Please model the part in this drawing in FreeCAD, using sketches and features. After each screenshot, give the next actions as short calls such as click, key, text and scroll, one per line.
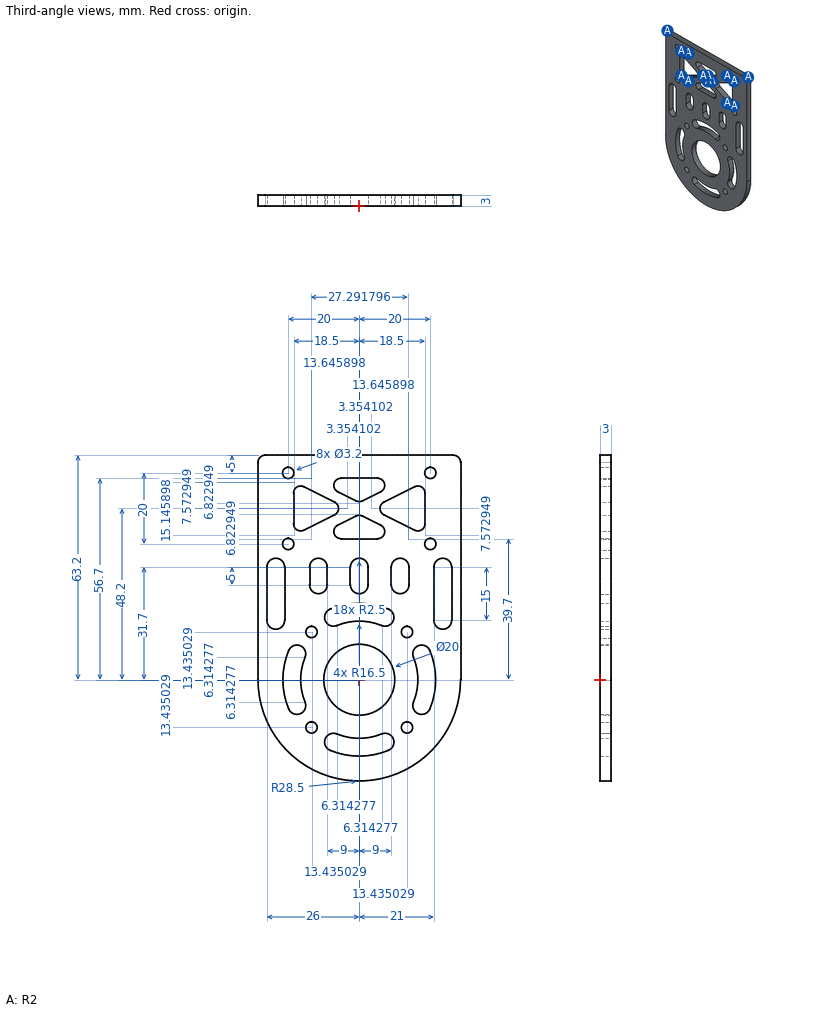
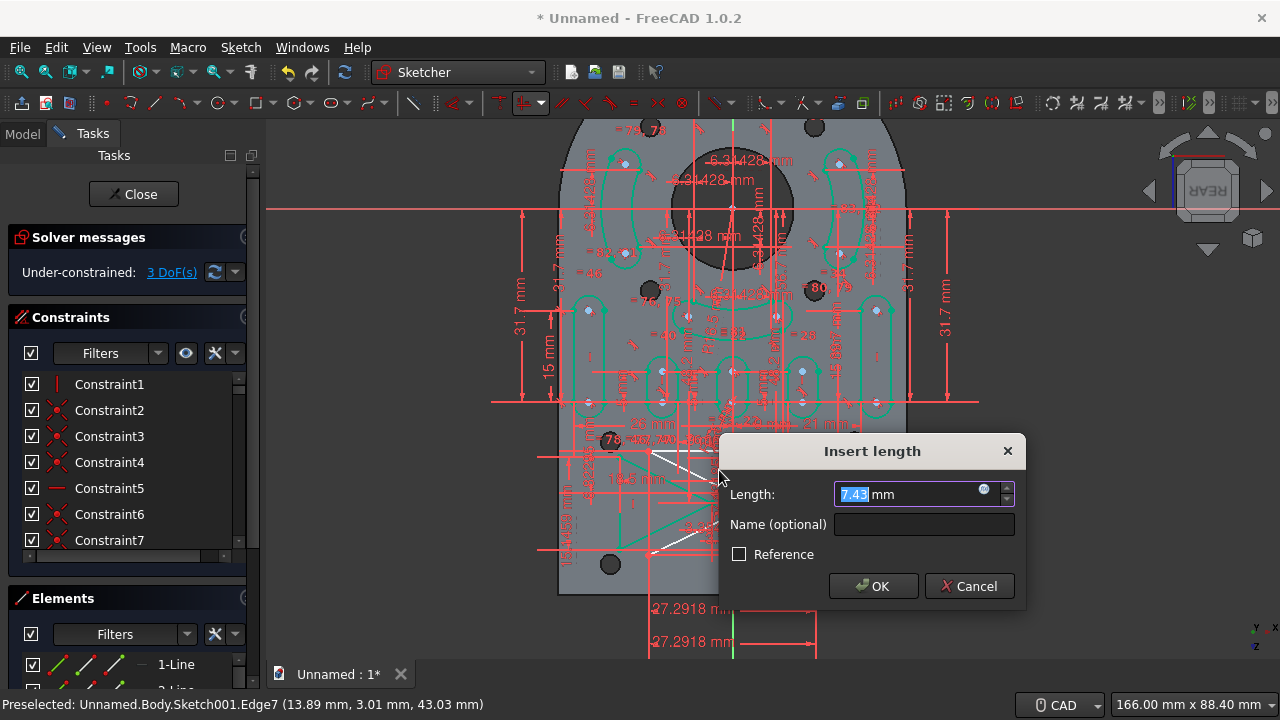
text(7.572949)
key(Return)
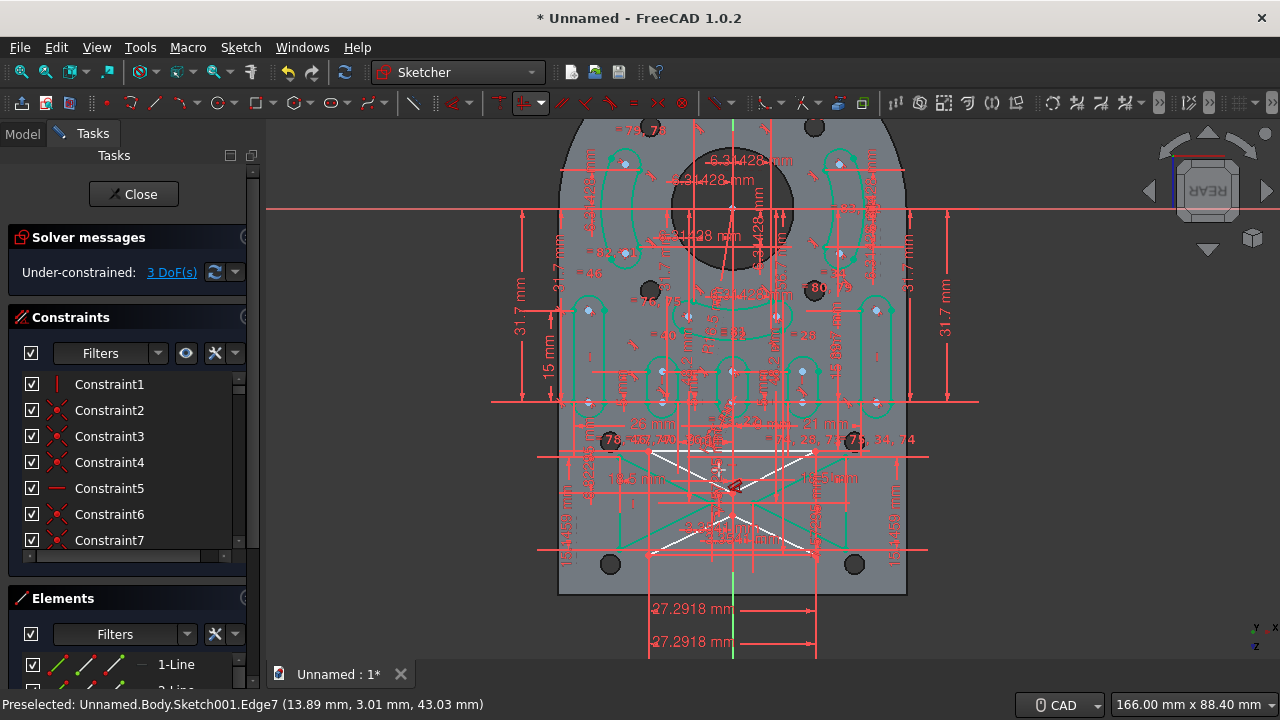
click(707, 527)
click(591, 549)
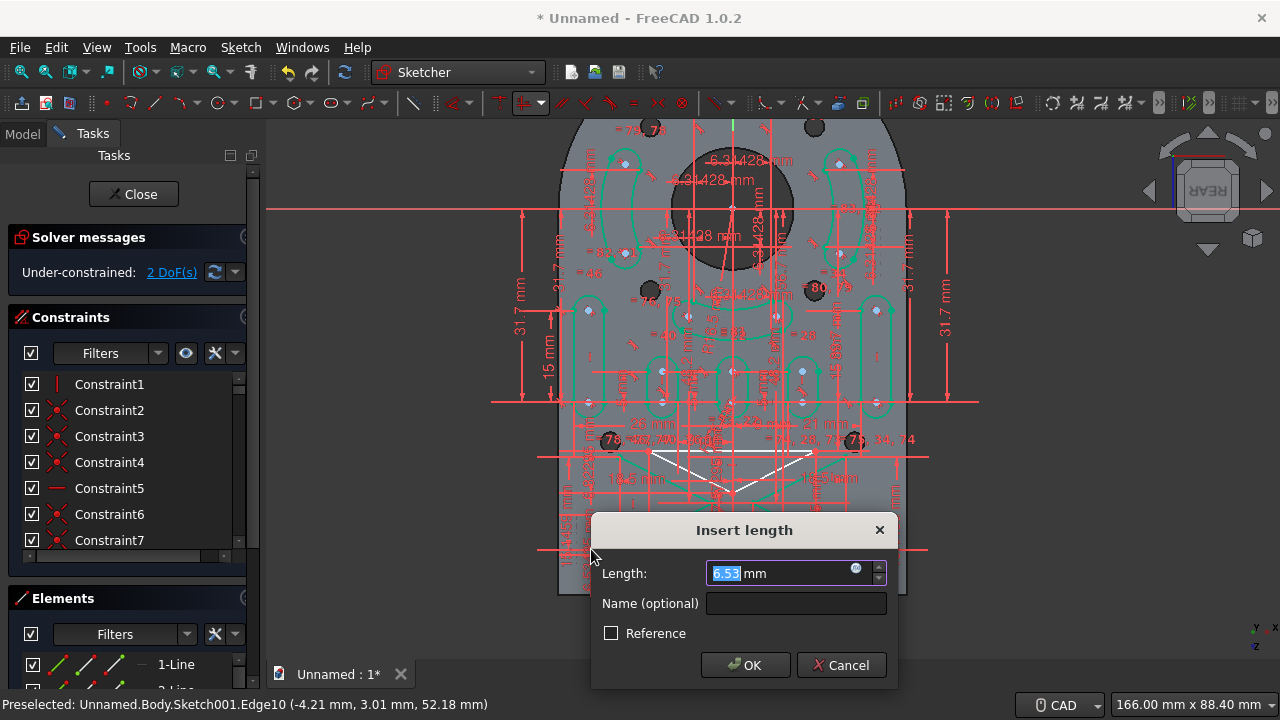
text(6.822949)
key(Return)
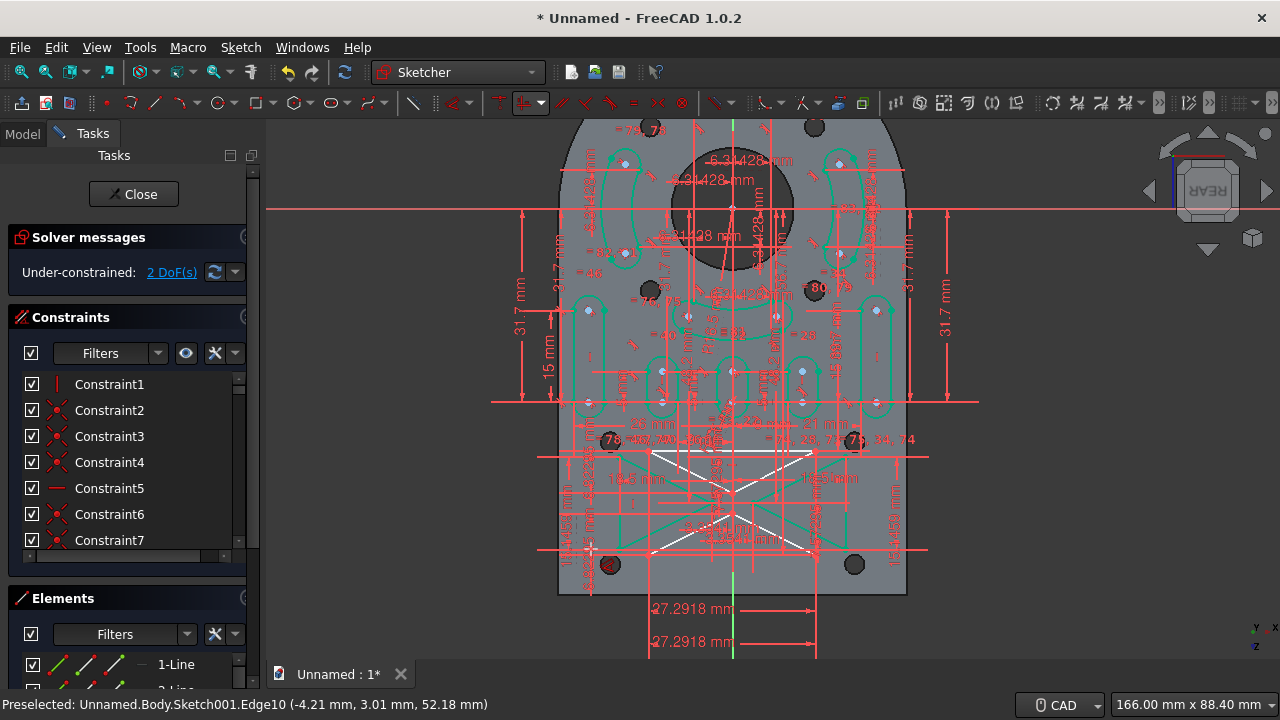
click(816, 451)
click(774, 581)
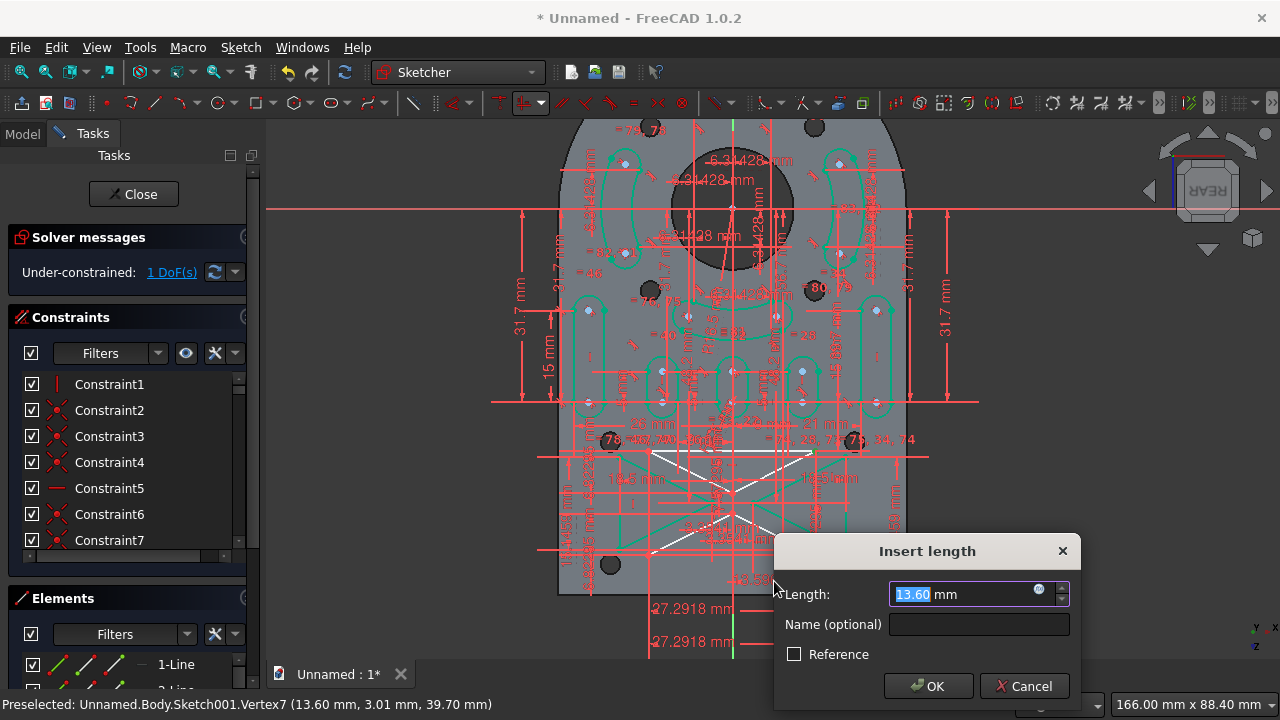
text(13.645898)
key(Return)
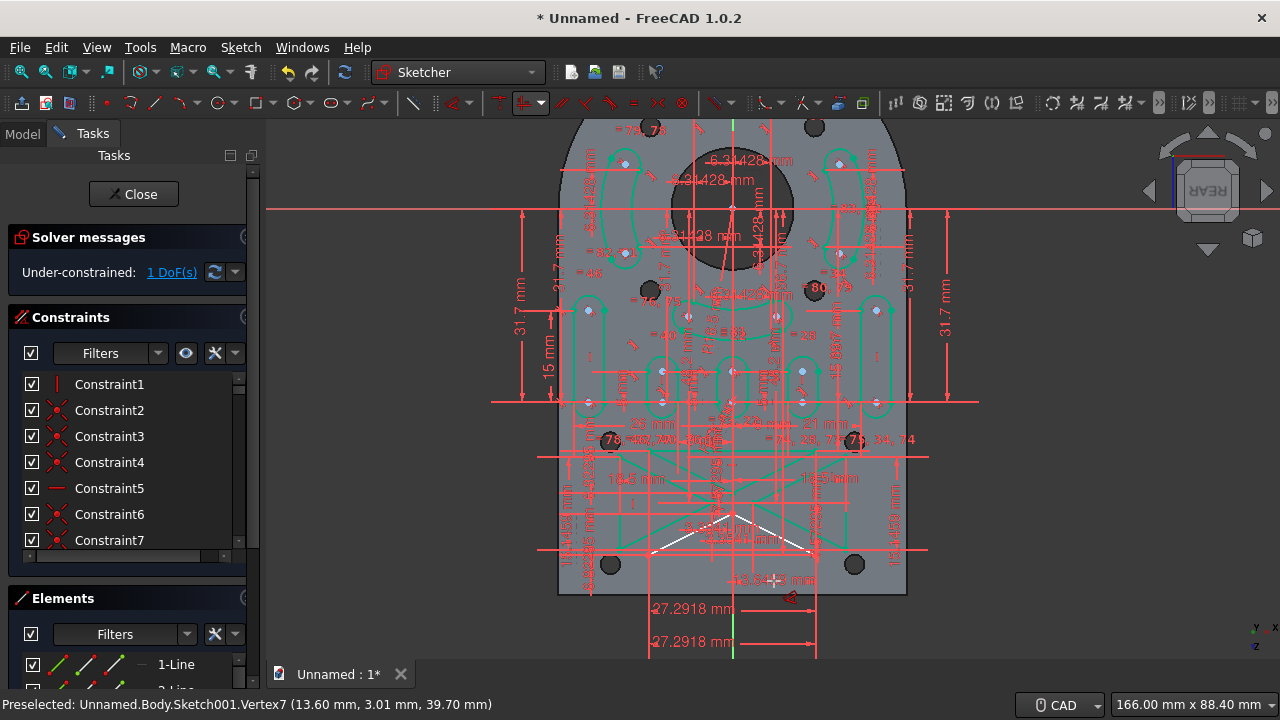
click(649, 555)
click(691, 589)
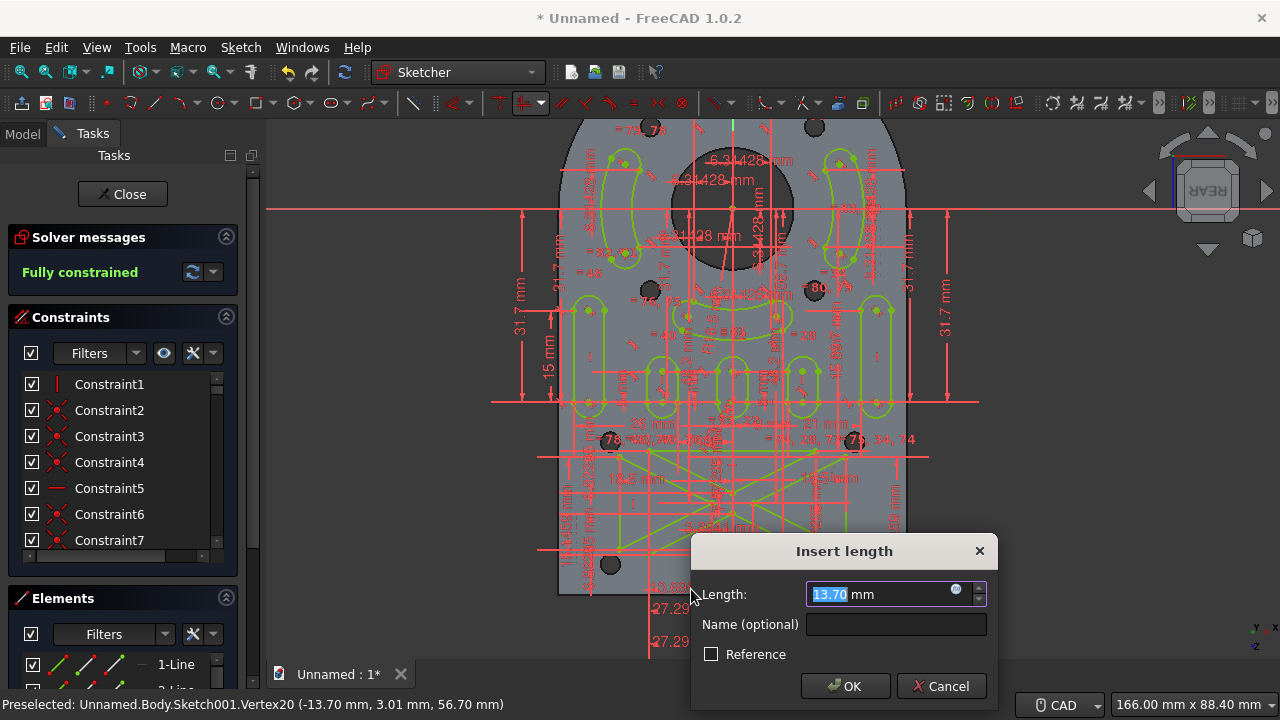
text(13.645898)
key(Return)
key(Escape)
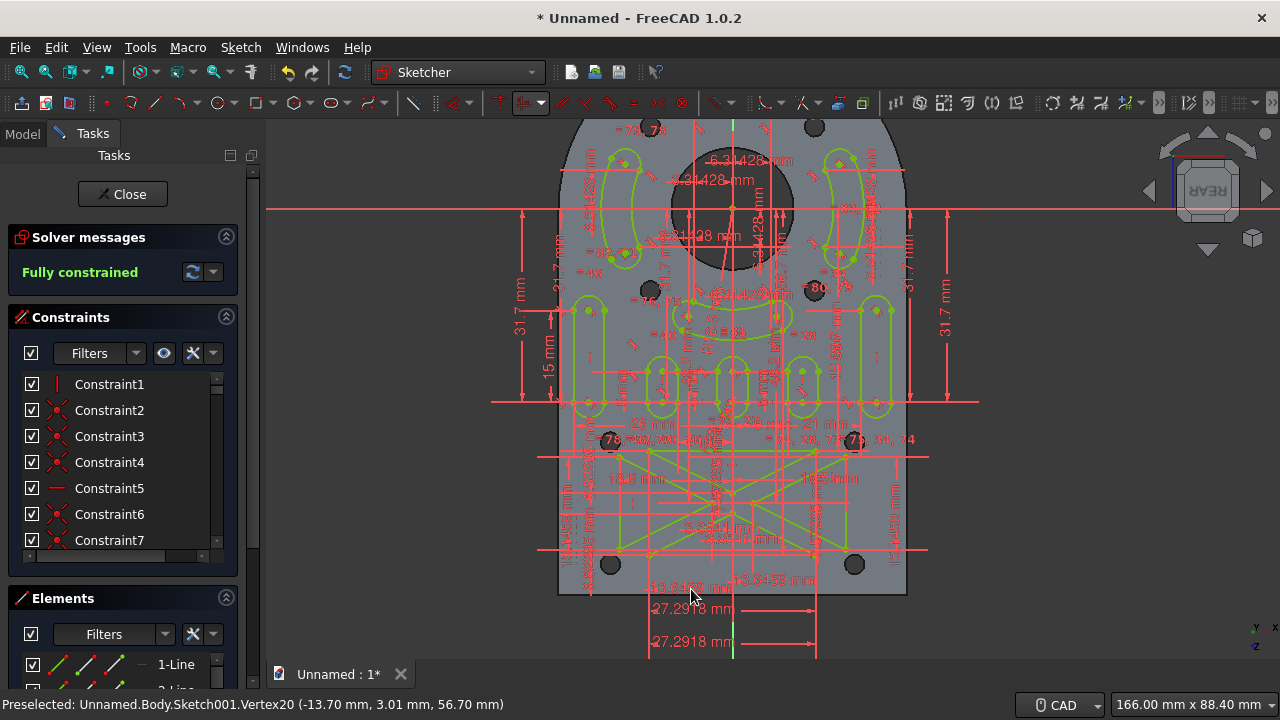
click(123, 194)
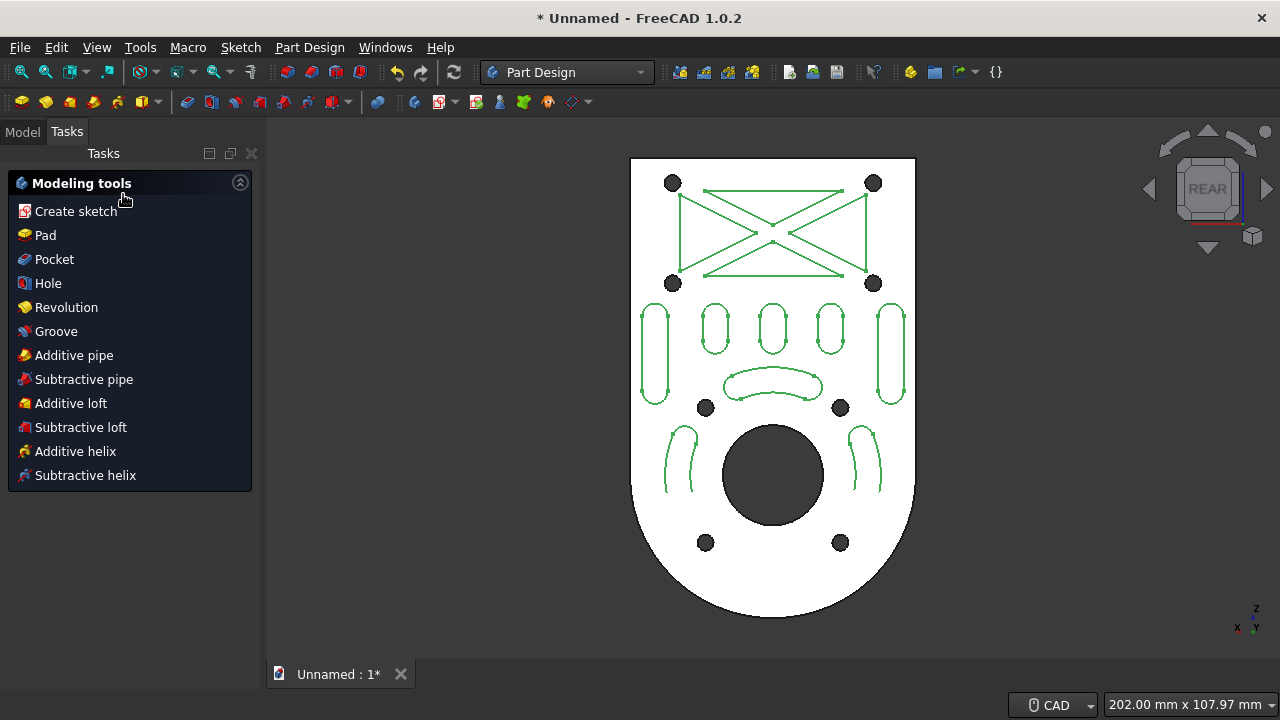
click(188, 102)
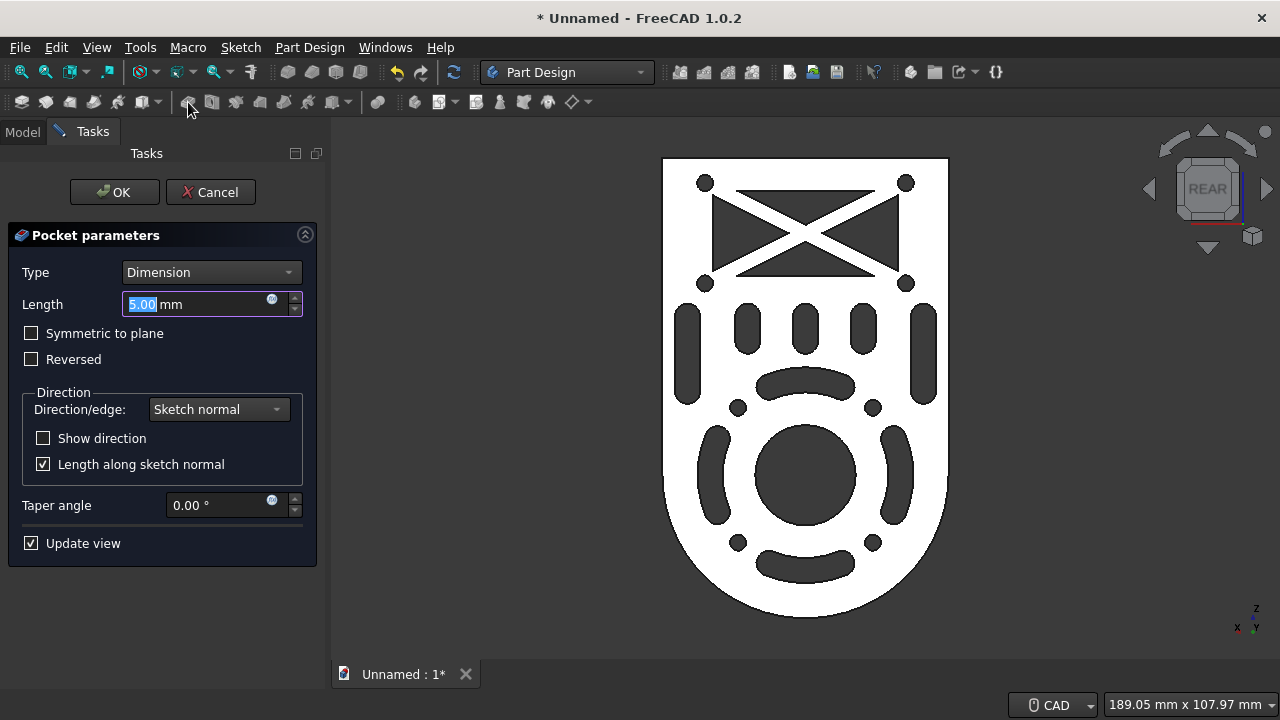
text(3)
key(Tab)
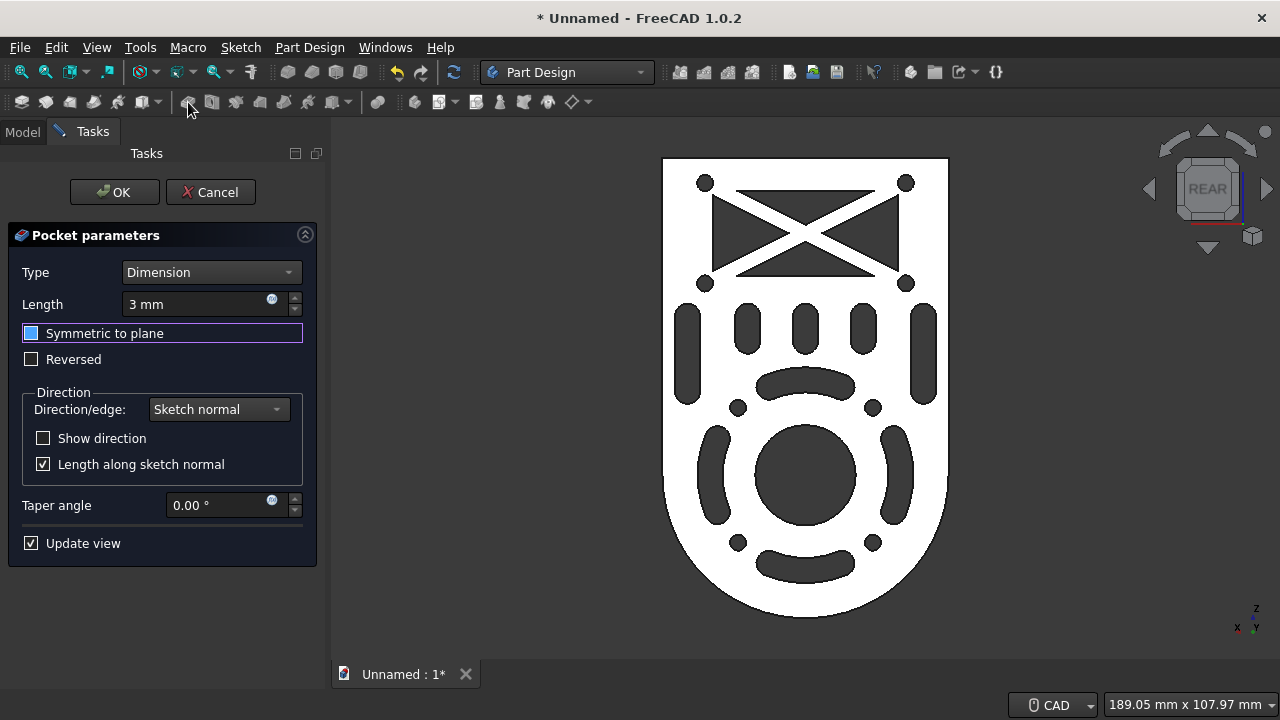
click(115, 192)